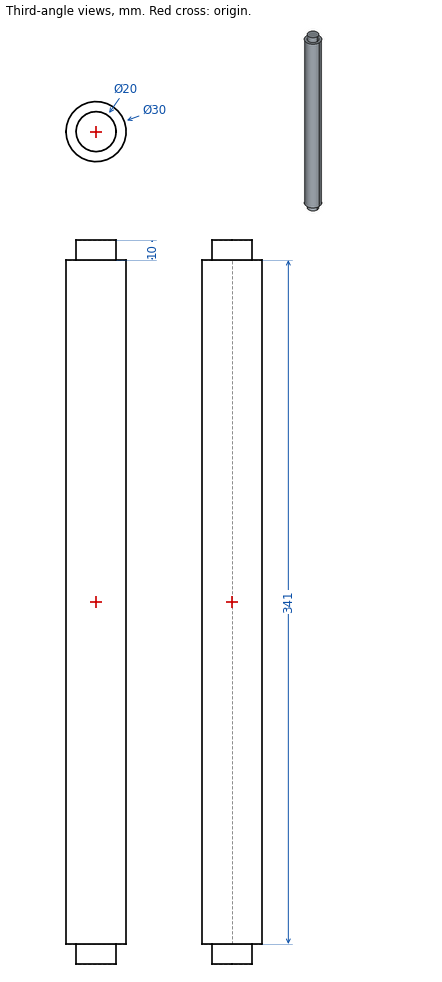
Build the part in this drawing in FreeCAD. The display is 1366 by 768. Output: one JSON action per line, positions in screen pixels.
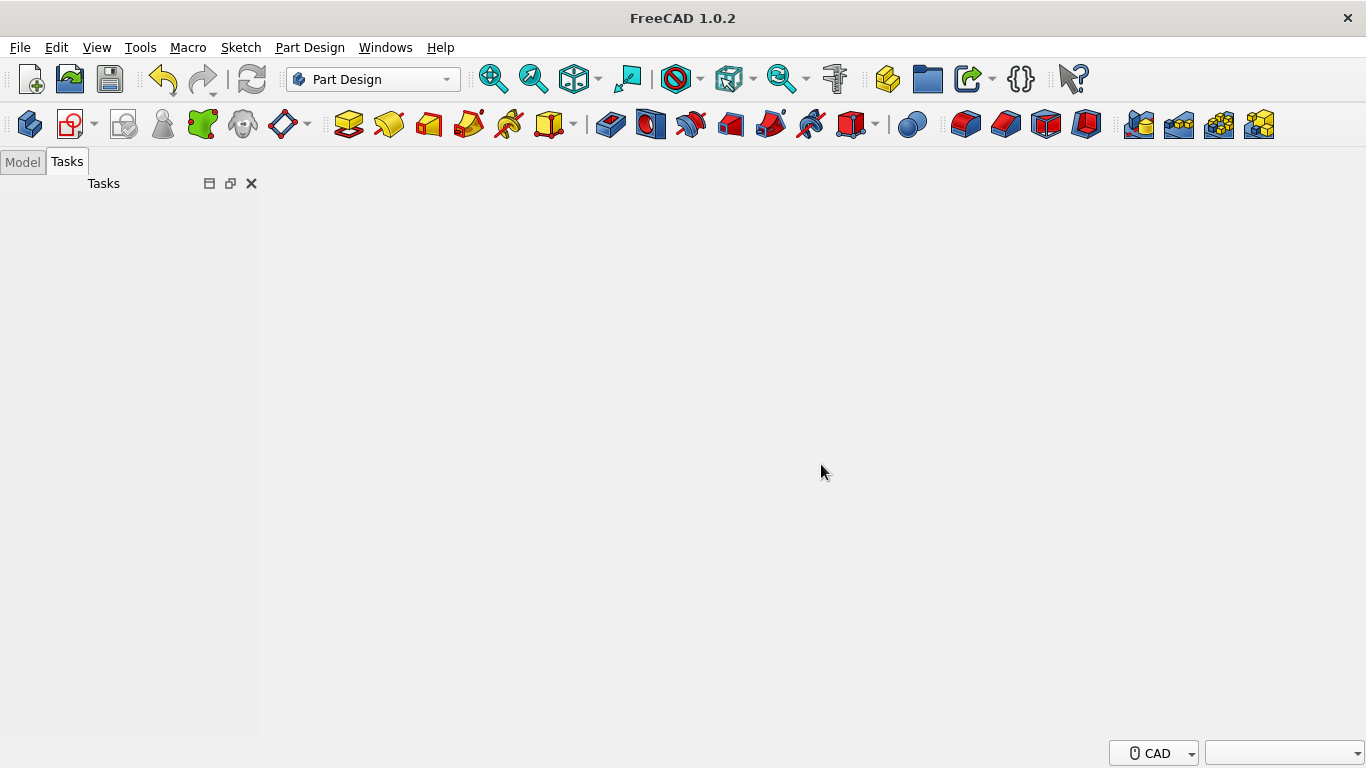
{"action": "left_click", "coordinate": [30, 80]}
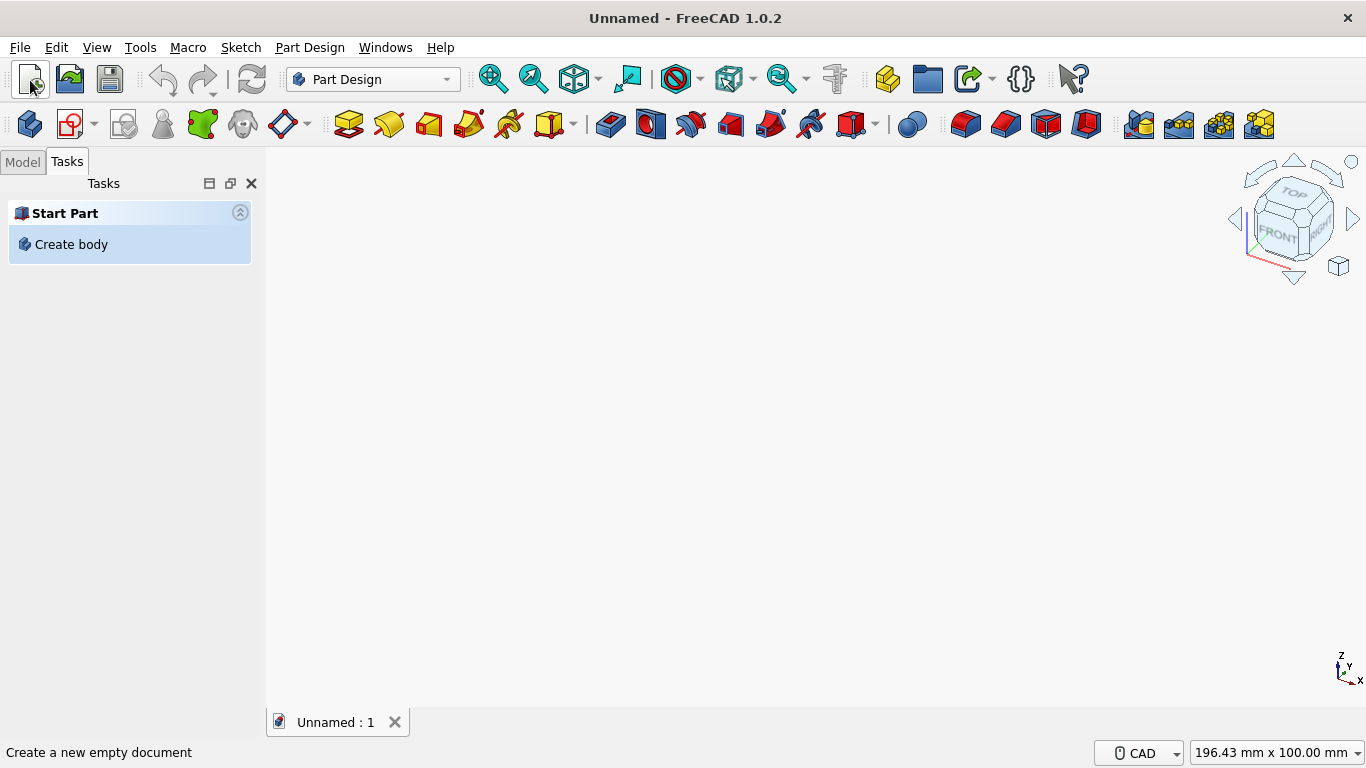
{"action": "left_click", "coordinate": [70, 124]}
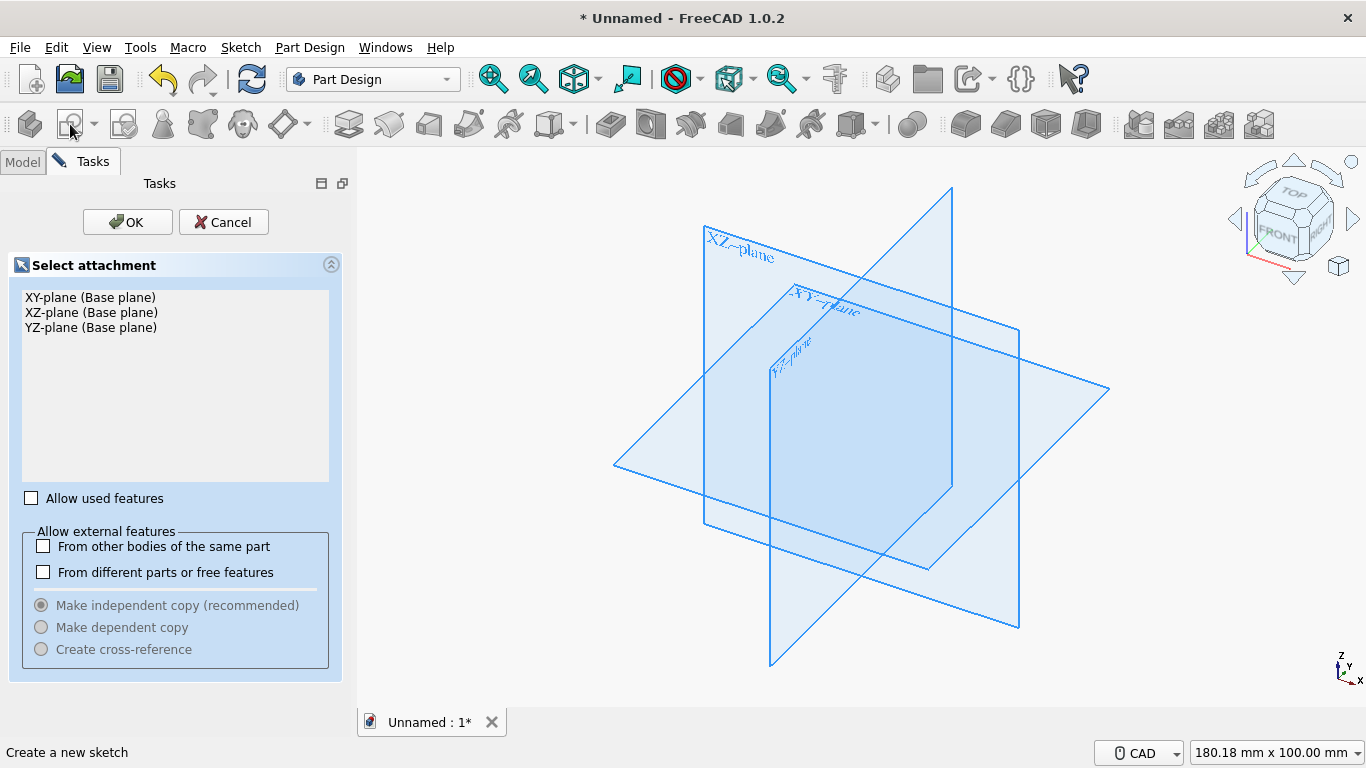
{"action": "left_click", "coordinate": [82, 298]}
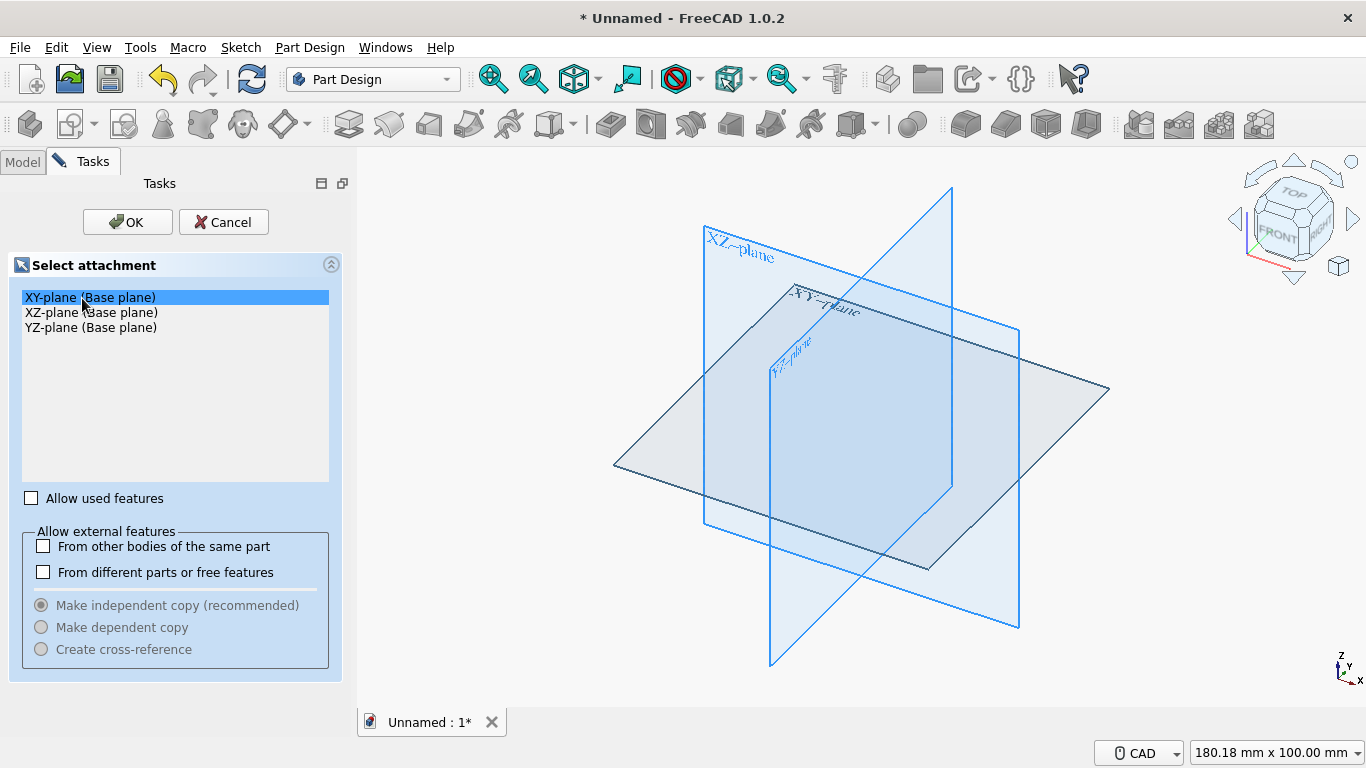
{"action": "left_click", "coordinate": [128, 222]}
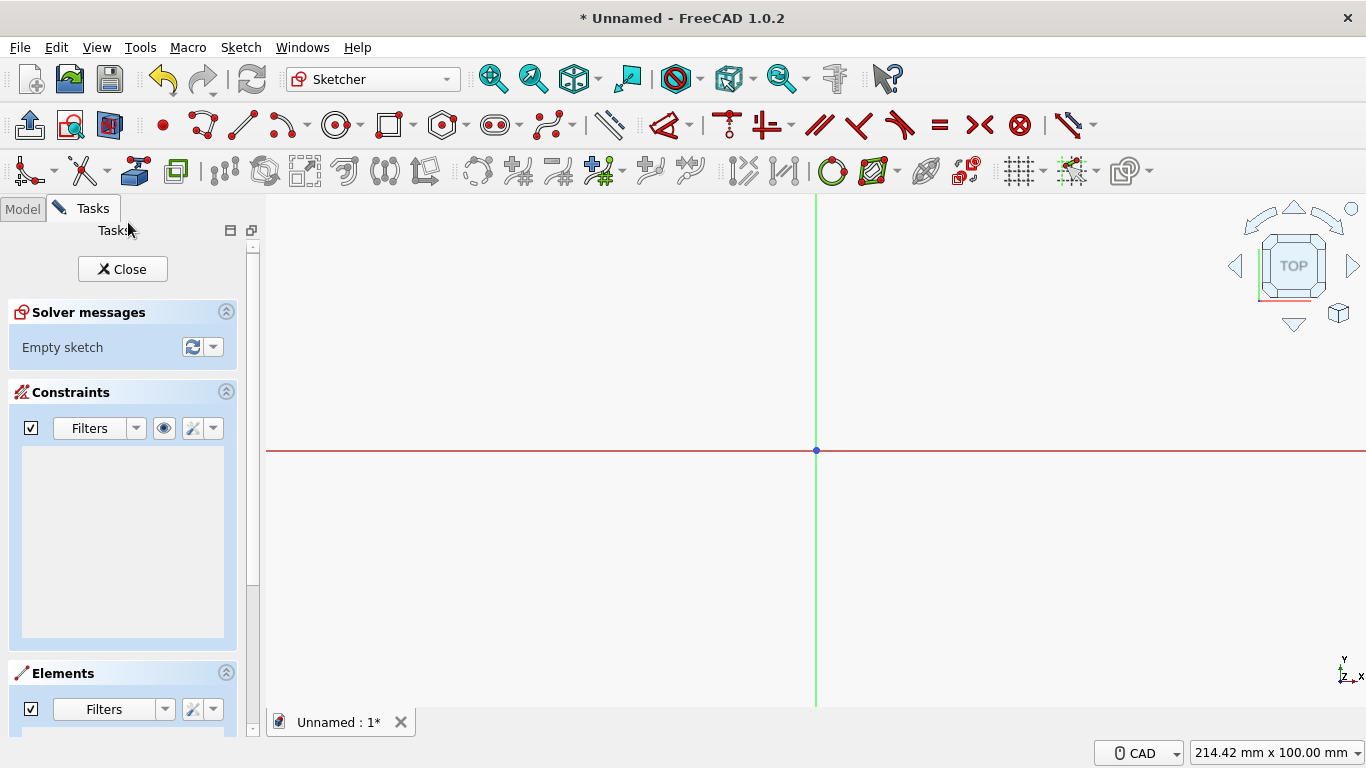
{"action": "scroll", "coordinate": [872, 450], "scroll_direction": "up", "scroll_amount": 4}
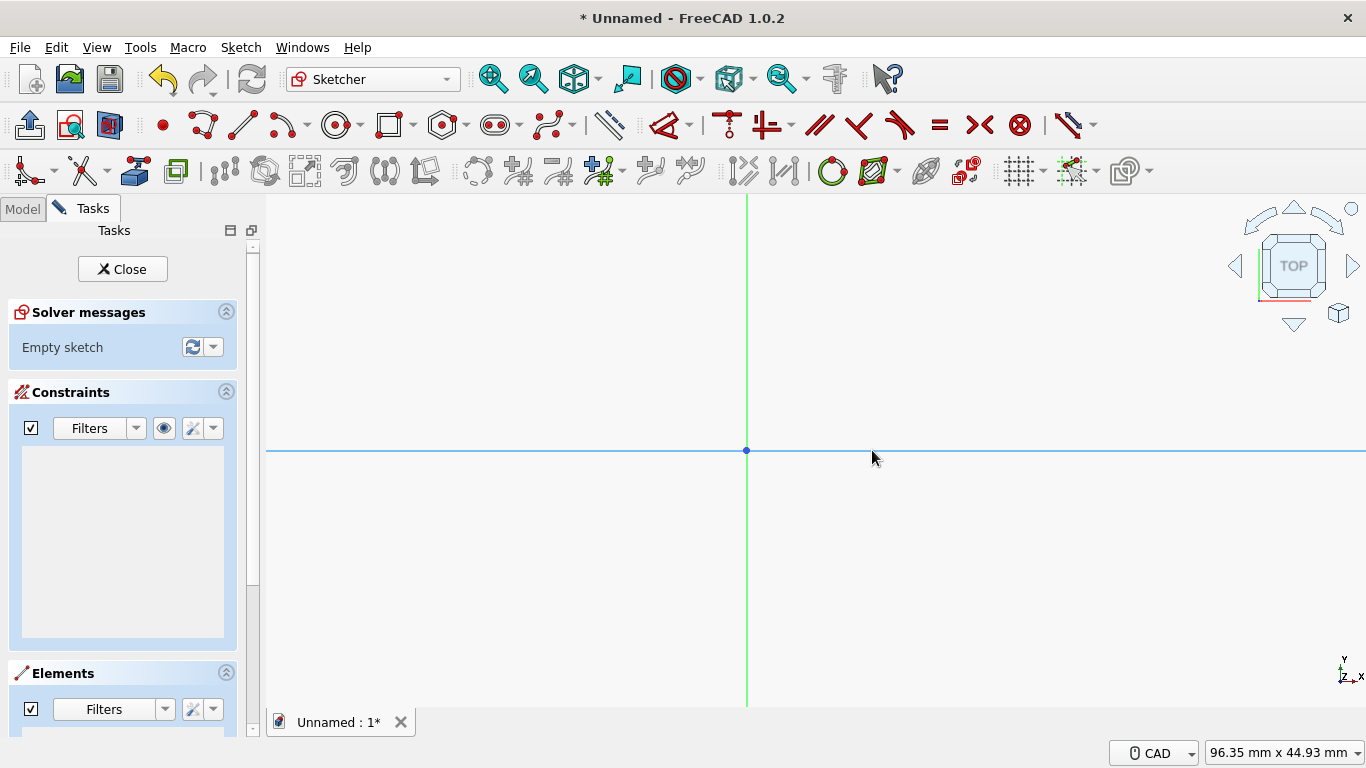
{"action": "left_click", "coordinate": [336, 126]}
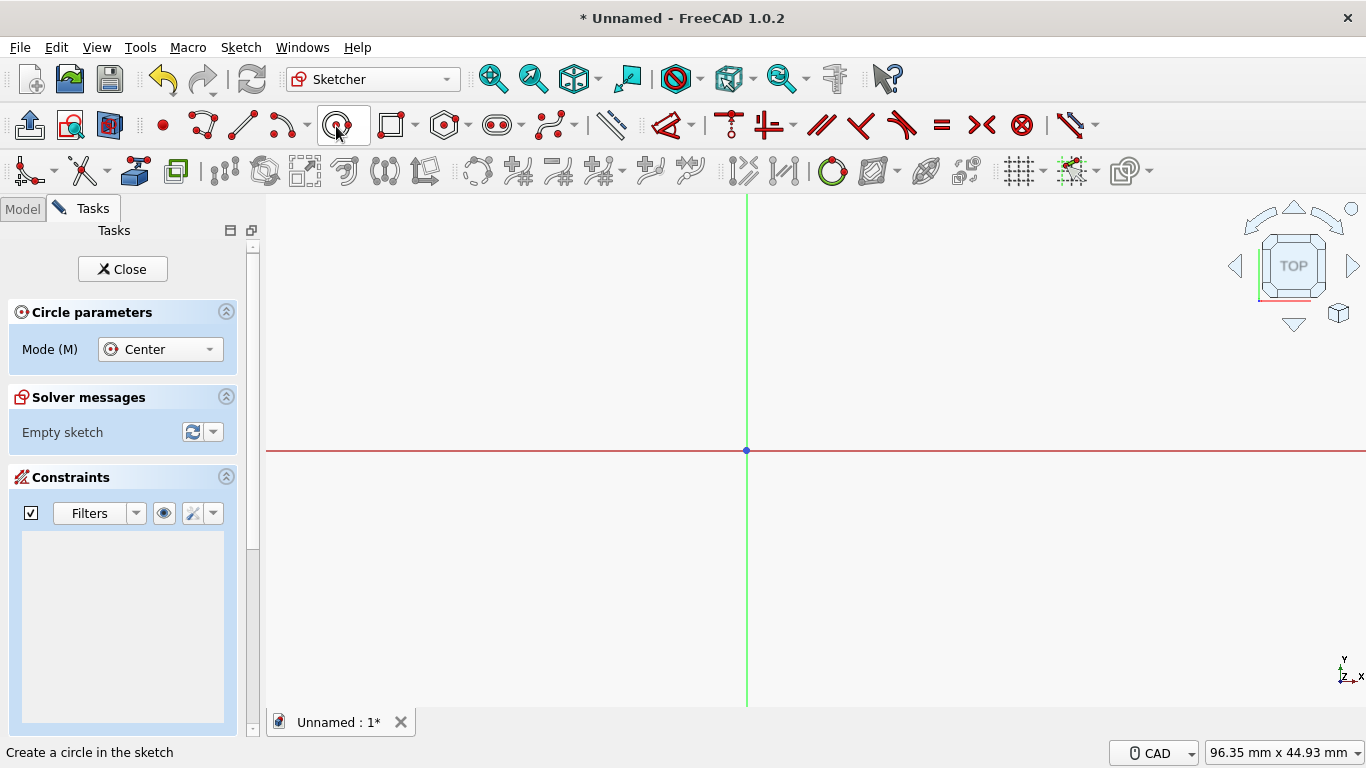
{"action": "left_click", "coordinate": [747, 450]}
{"action": "mouse_move", "coordinate": [868, 329]}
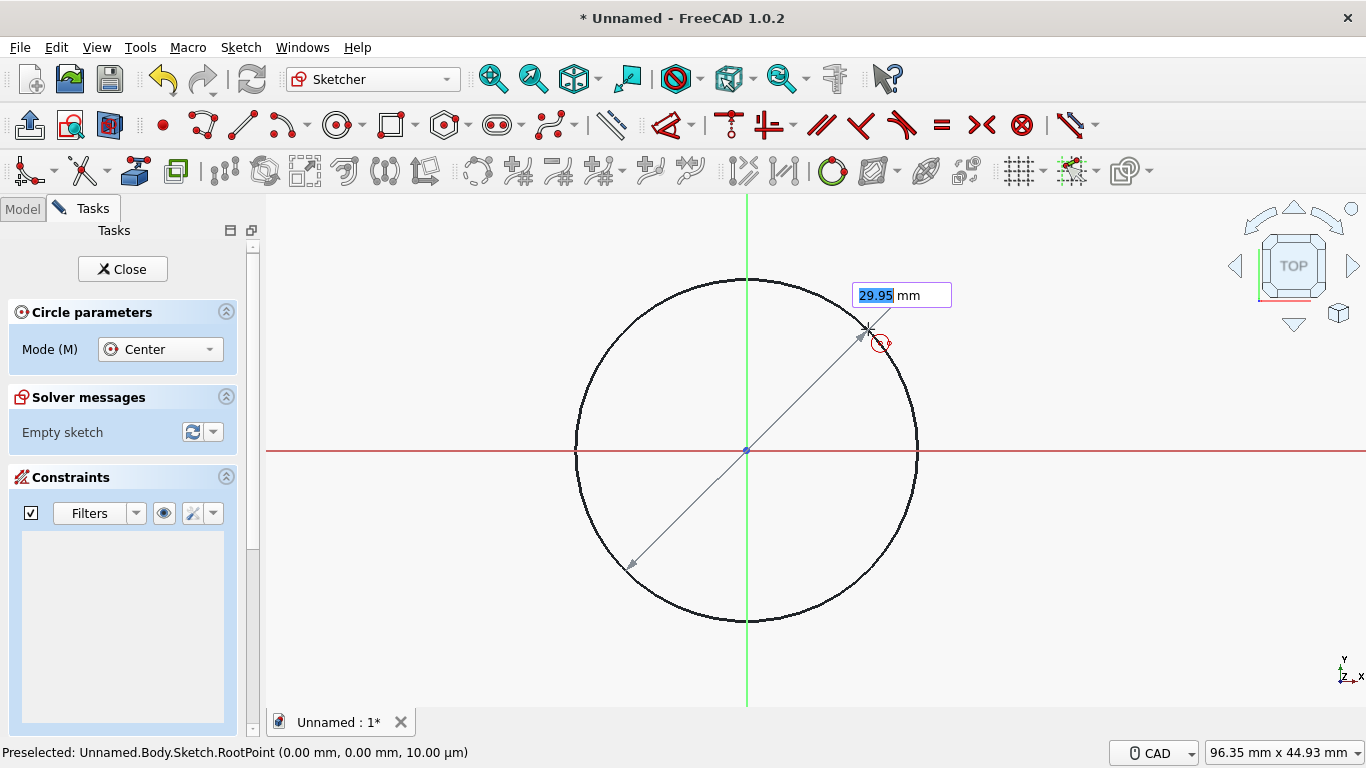
{"action": "type", "text": "30"}
{"action": "key", "text": "Return"}
{"action": "key", "text": "Escape"}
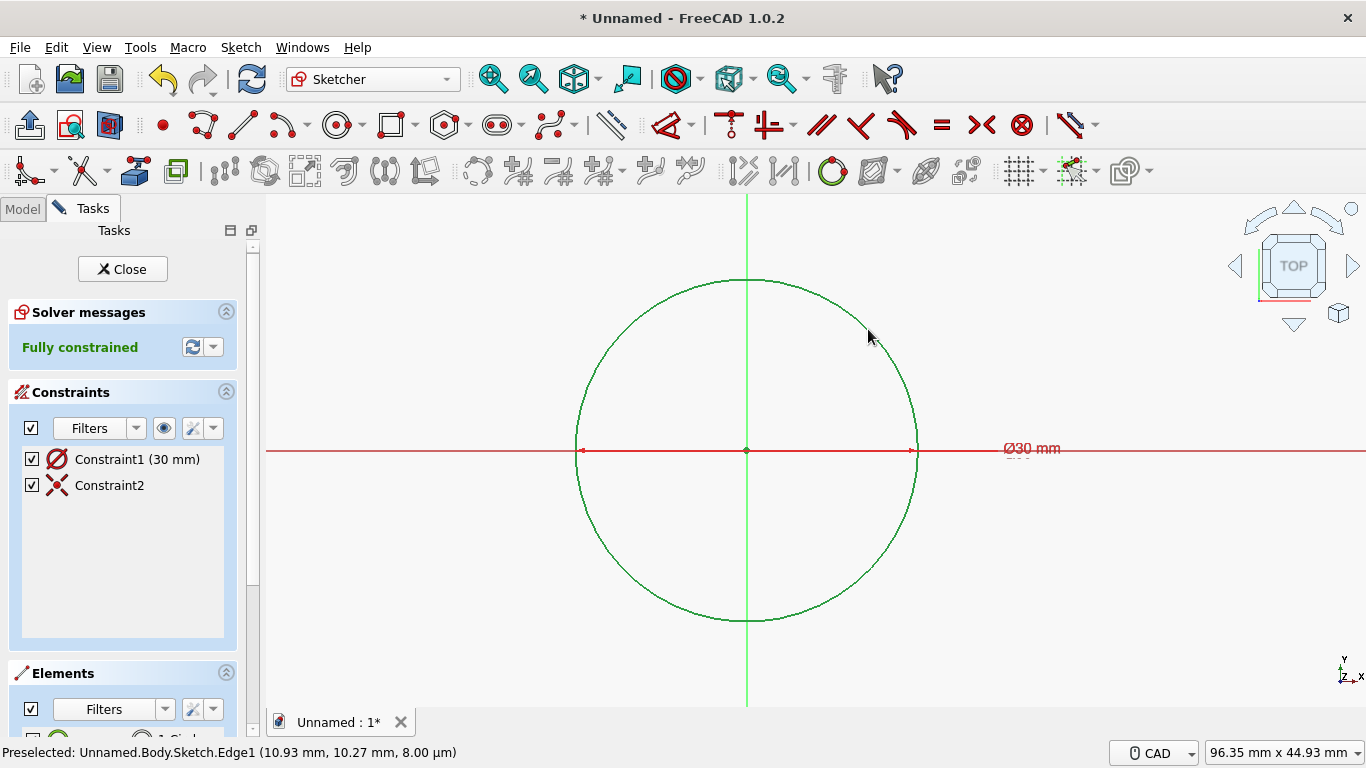
{"action": "left_click", "coordinate": [123, 269]}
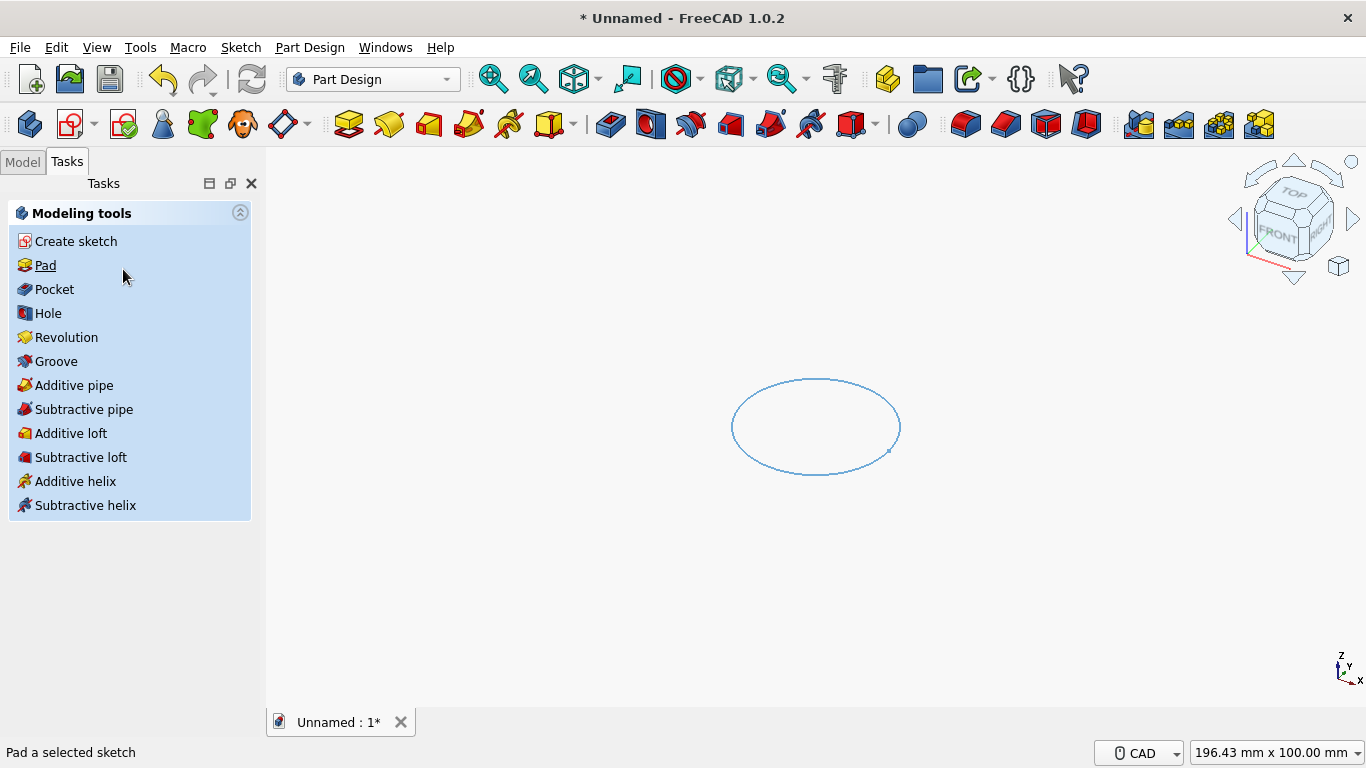
{"action": "left_click", "coordinate": [350, 124]}